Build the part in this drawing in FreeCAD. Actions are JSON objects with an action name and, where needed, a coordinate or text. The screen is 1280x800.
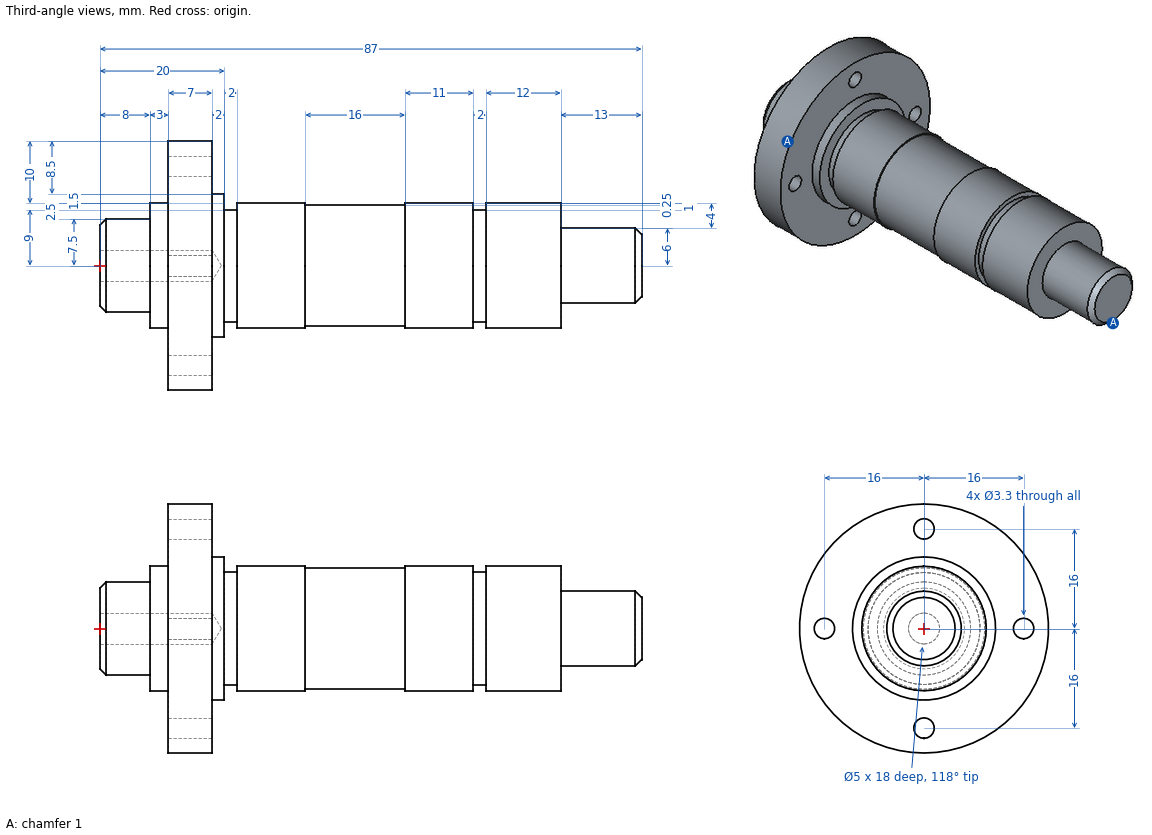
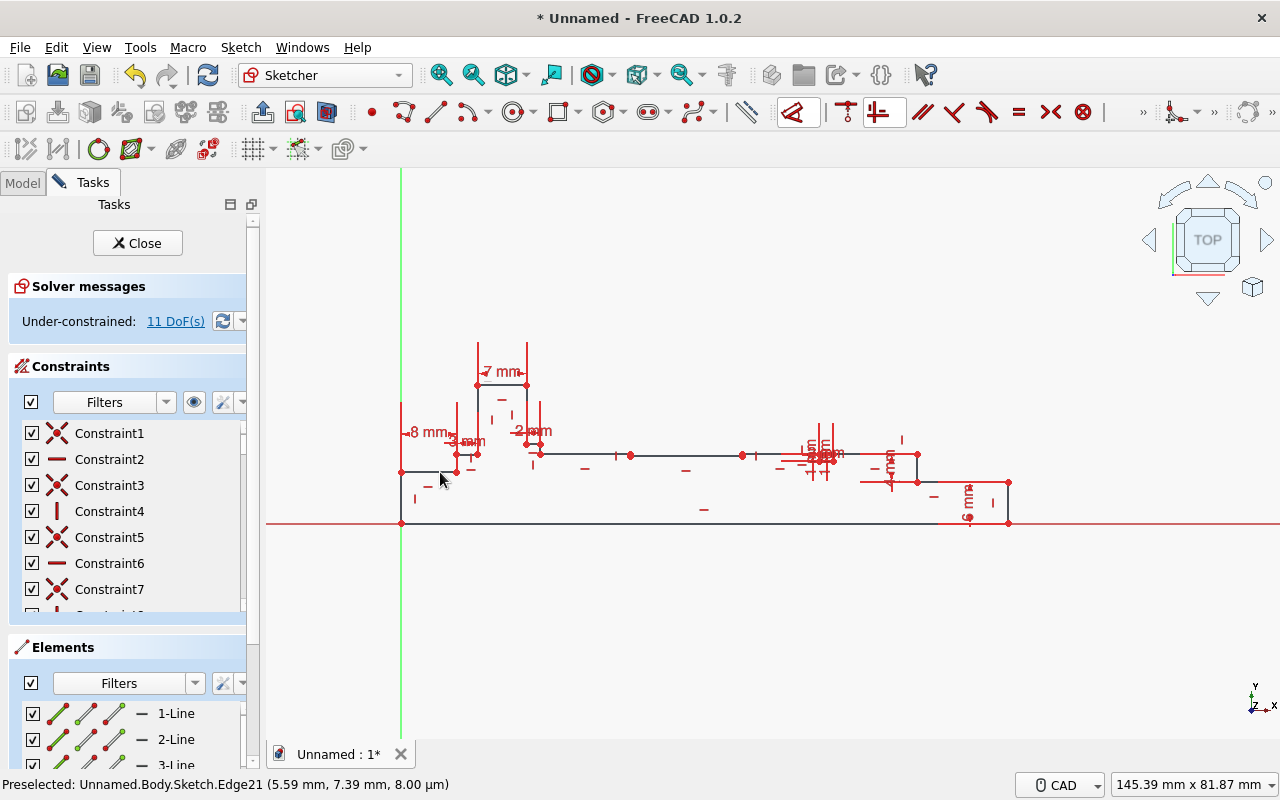
{"action": "left_click", "coordinate": [583, 524]}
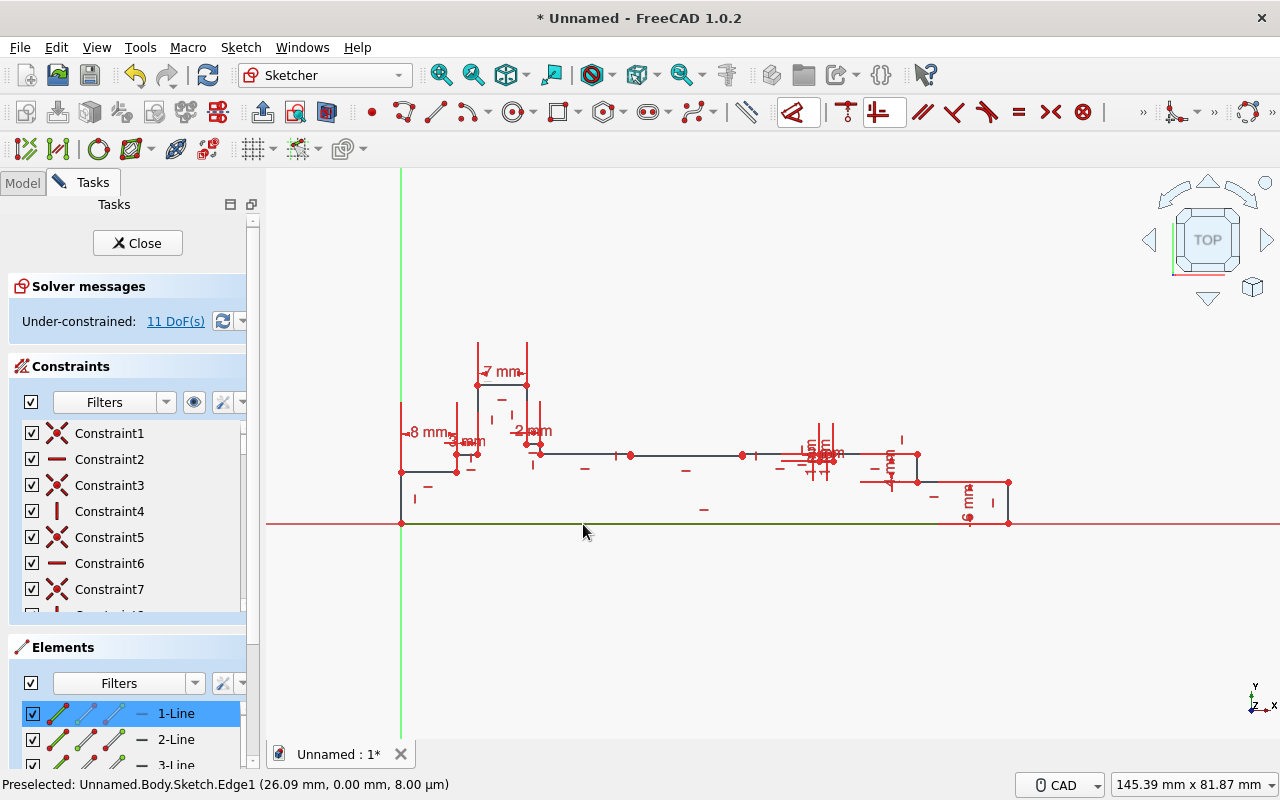
{"action": "left_click", "coordinate": [814, 112]}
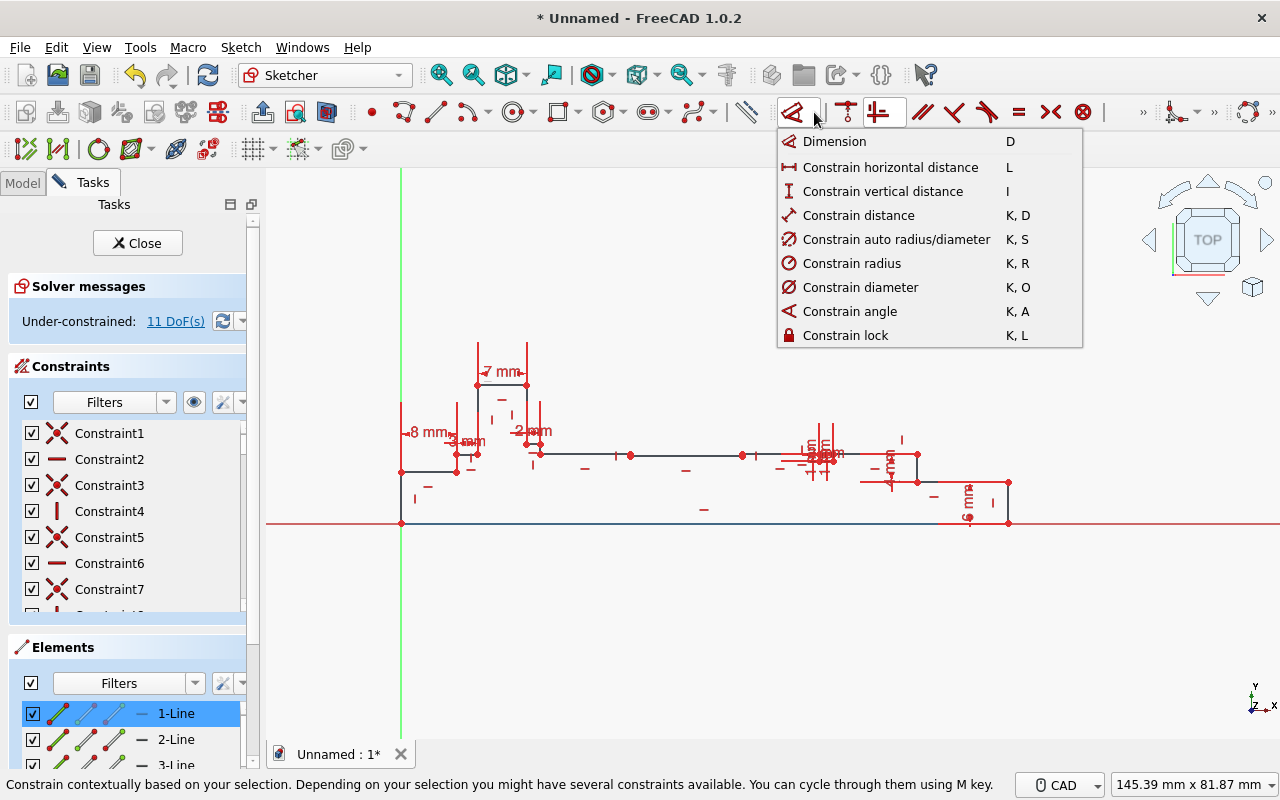
{"action": "left_click", "coordinate": [930, 167]}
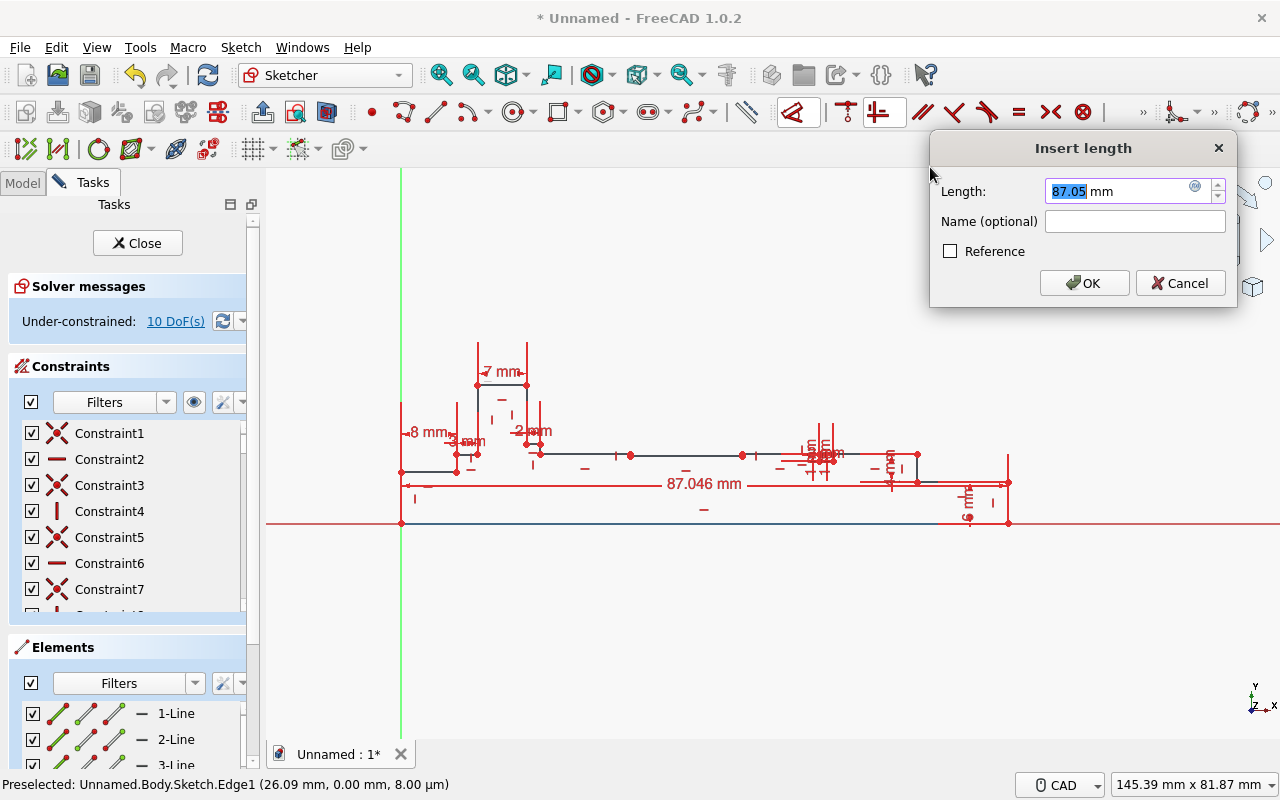
{"action": "type", "text": "87"}
{"action": "key", "text": "Return"}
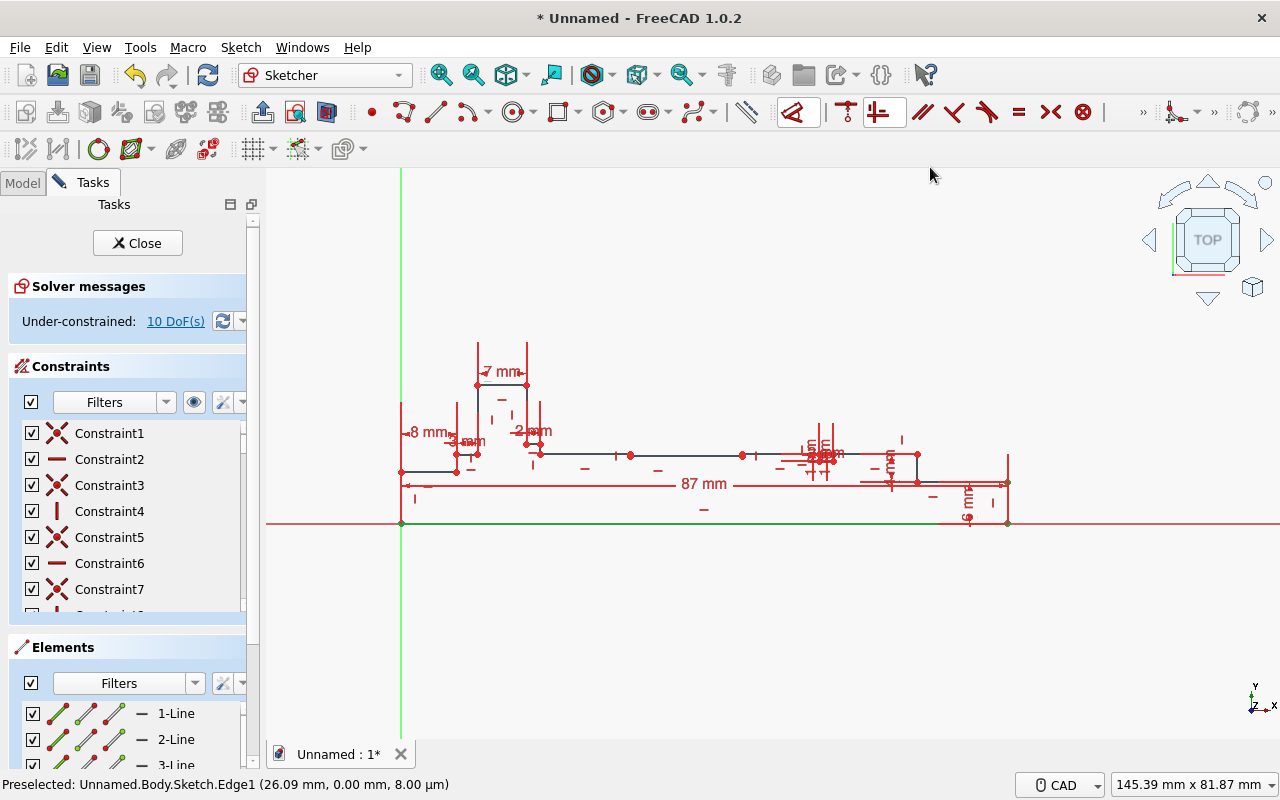
{"action": "left_click", "coordinate": [981, 482]}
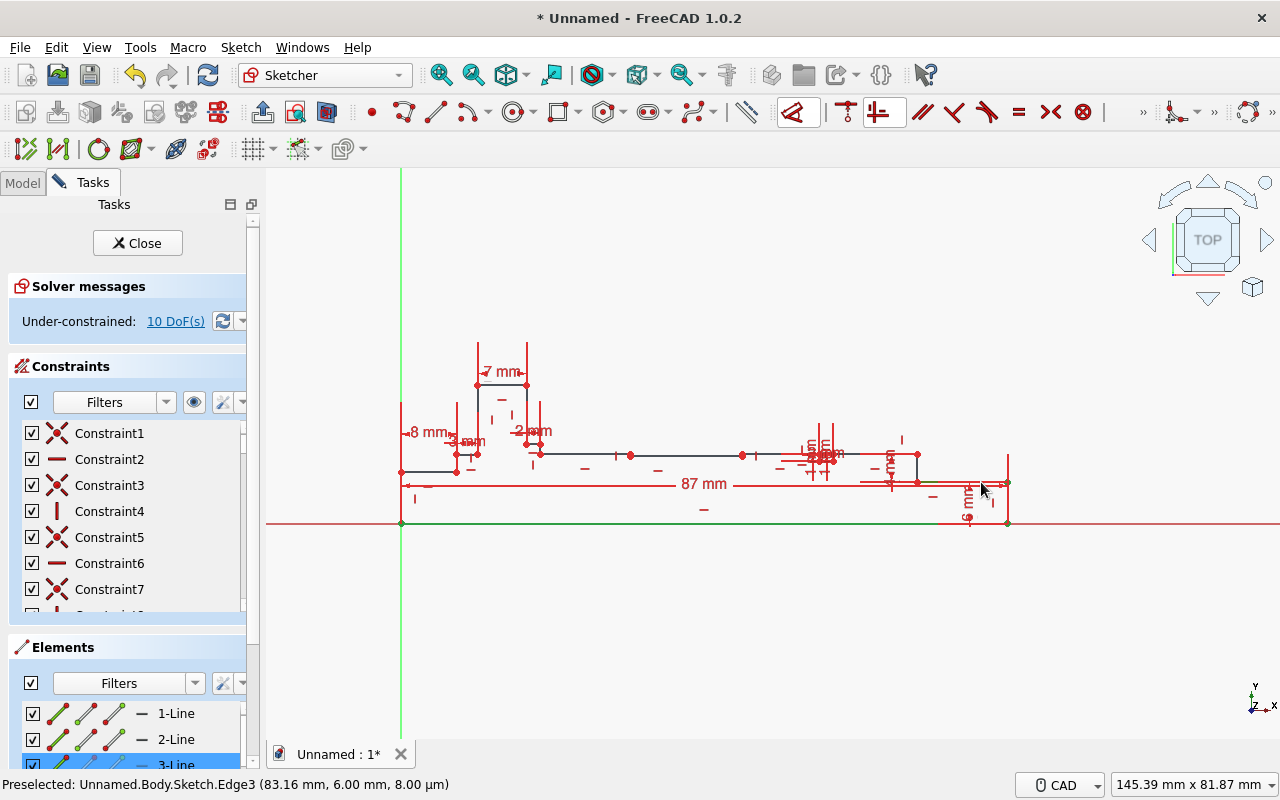
{"action": "left_click", "coordinate": [814, 112]}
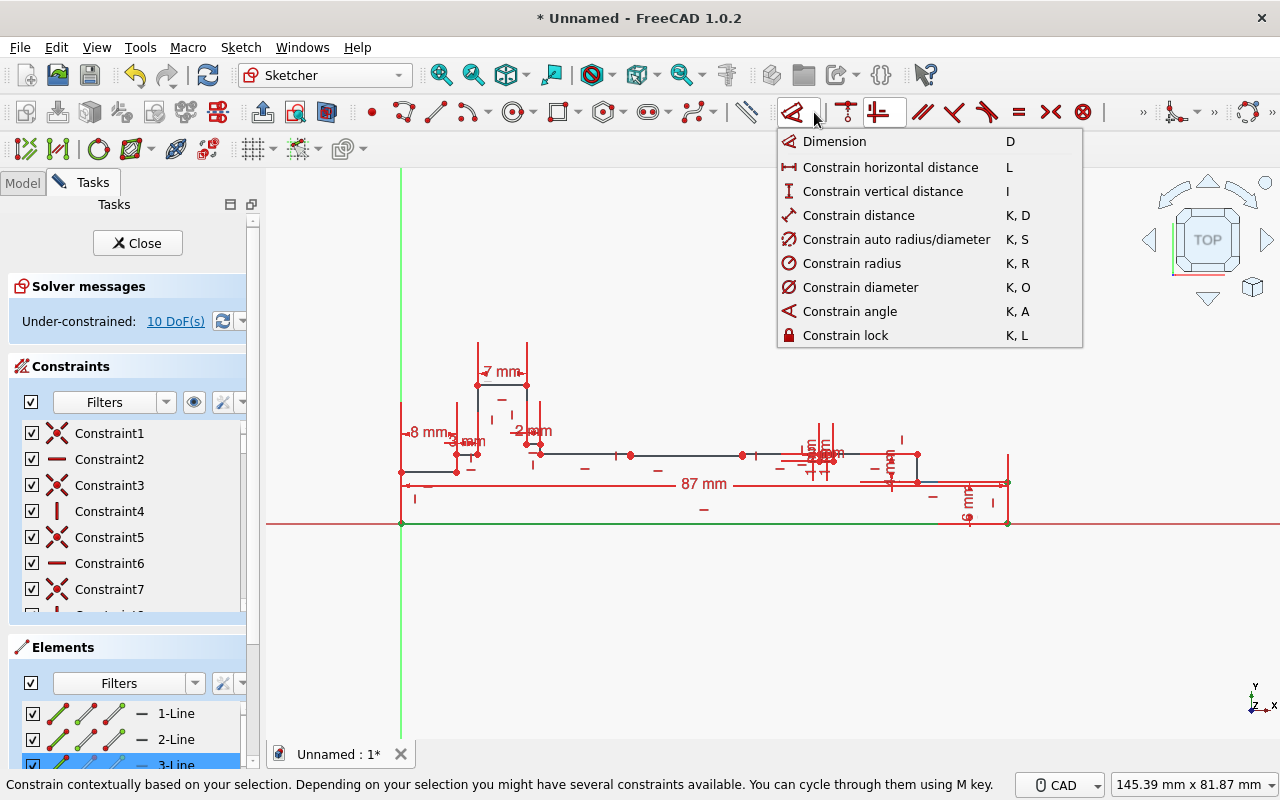
{"action": "left_click", "coordinate": [930, 167]}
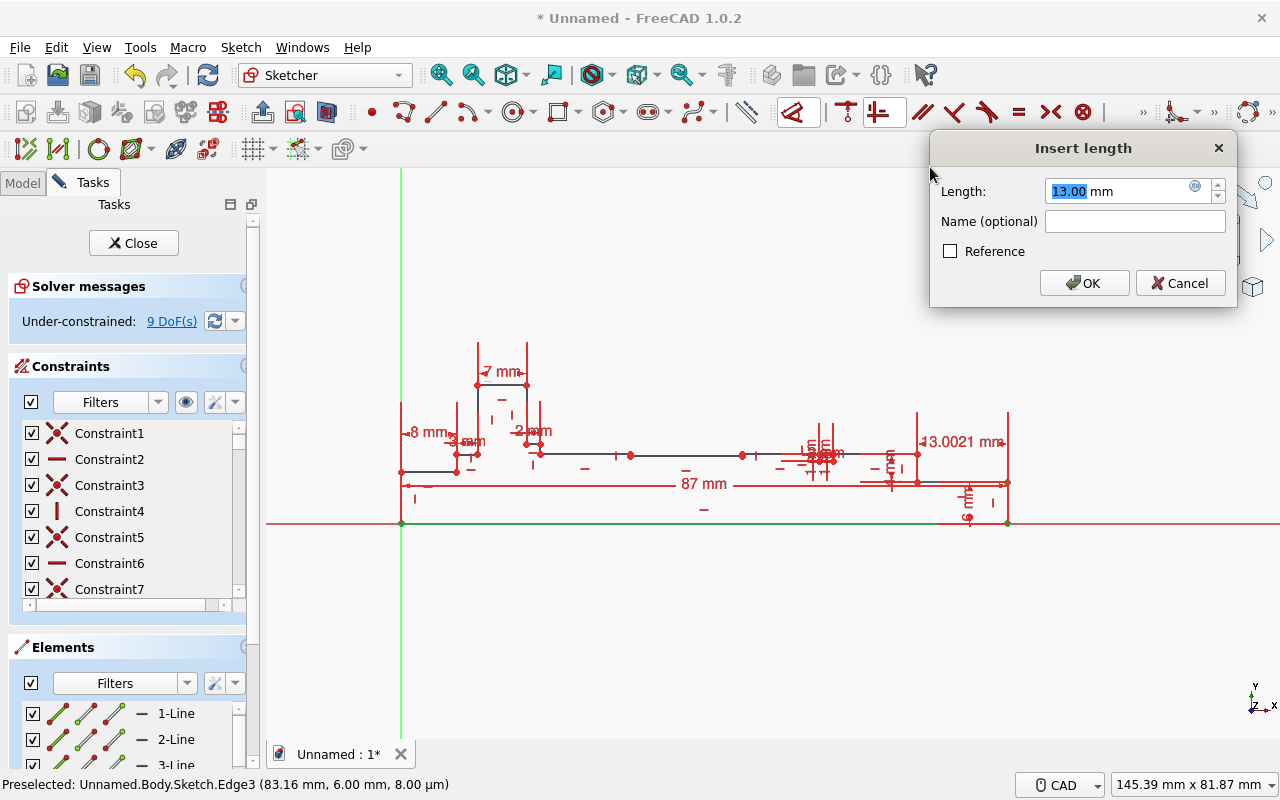
{"action": "type", "text": "13"}
{"action": "key", "text": "Return"}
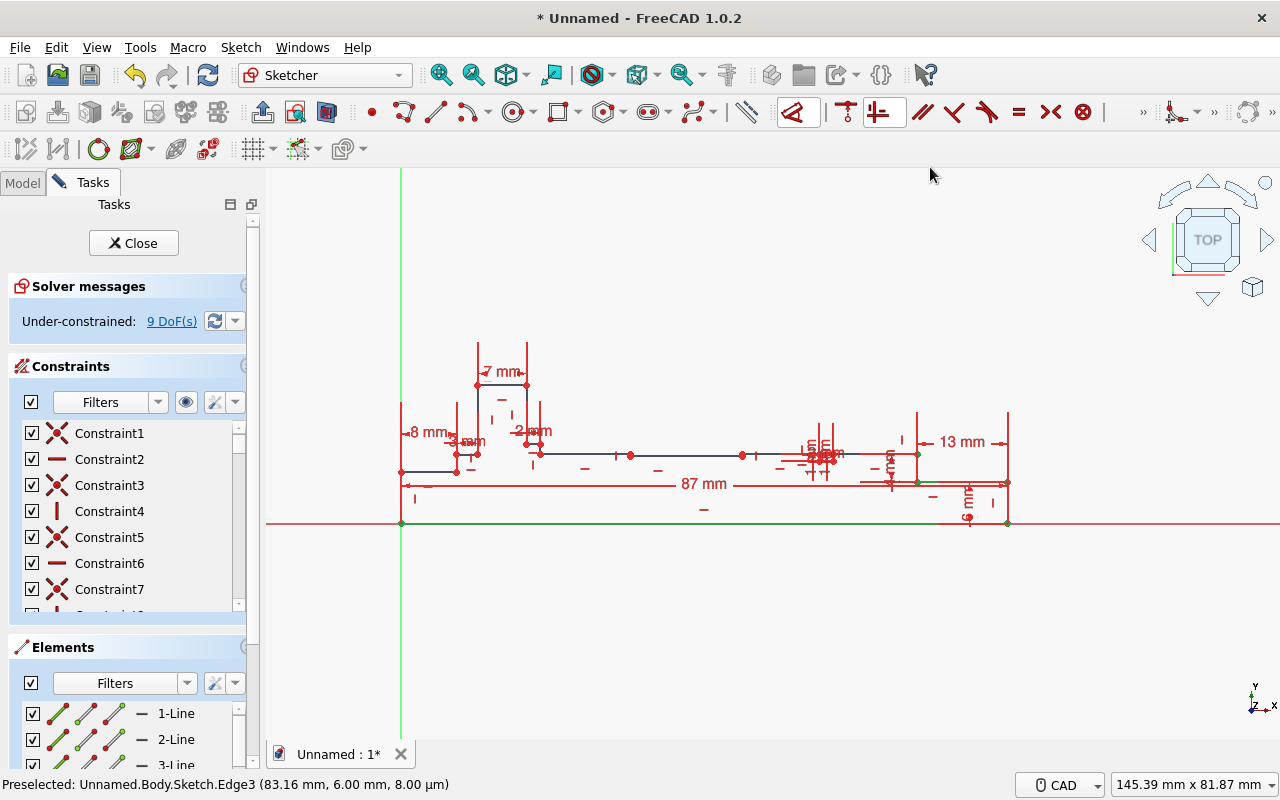
{"action": "left_click", "coordinate": [858, 454]}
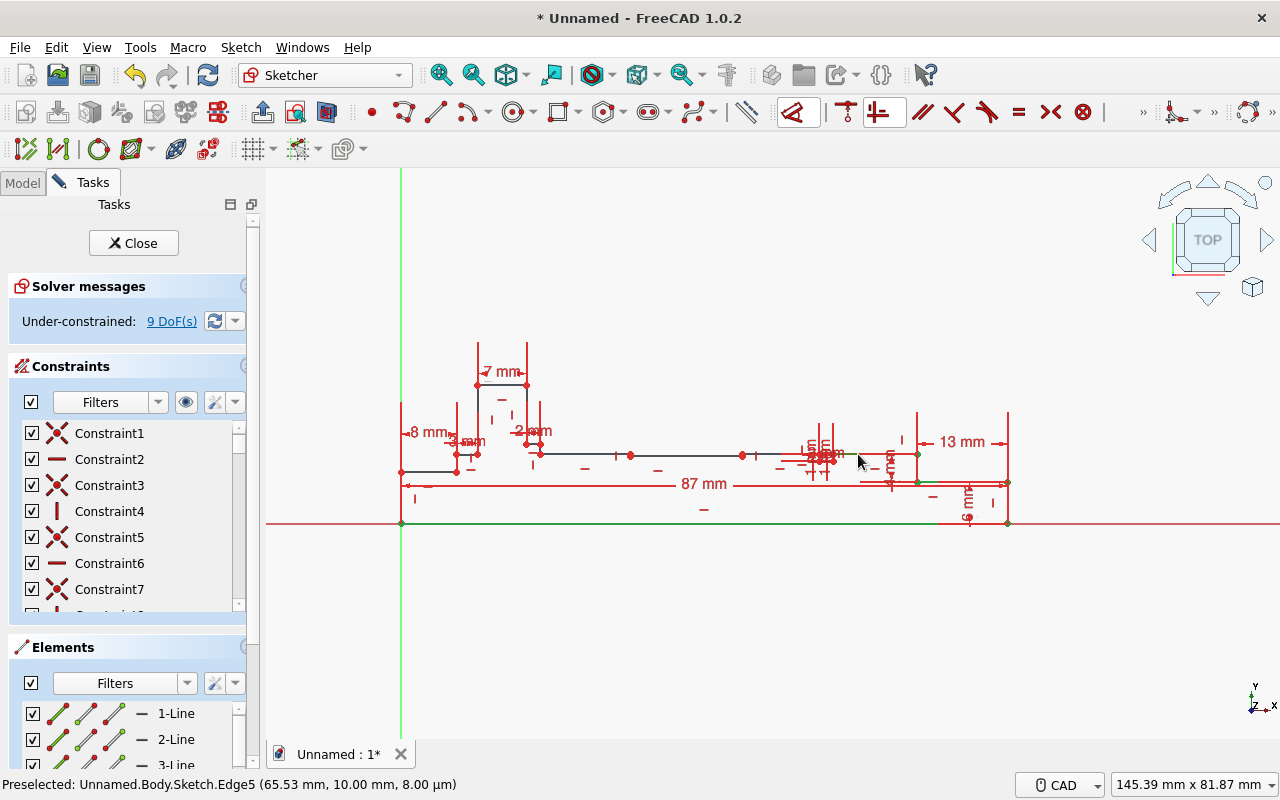
{"action": "key", "text": "l"}